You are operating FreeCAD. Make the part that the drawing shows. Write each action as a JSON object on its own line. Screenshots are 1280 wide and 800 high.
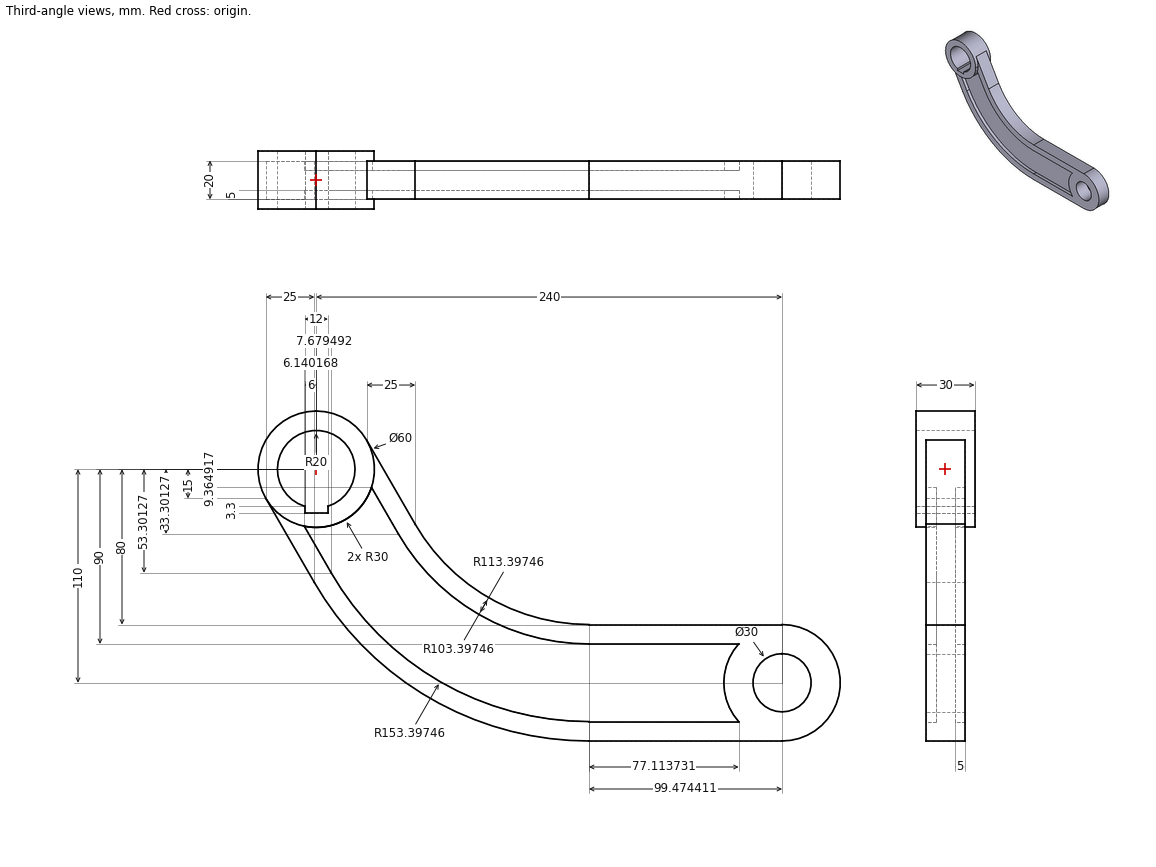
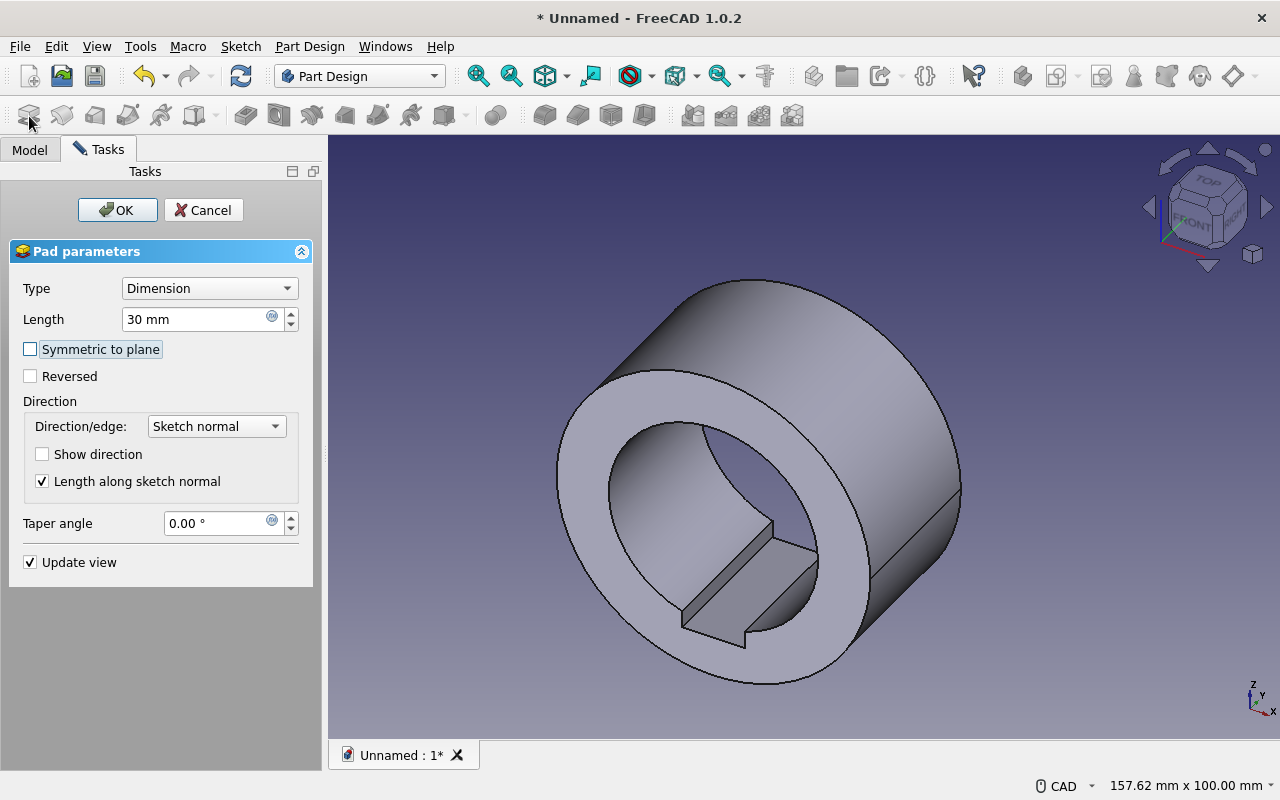
{"action": "left_click", "coordinate": [31, 349]}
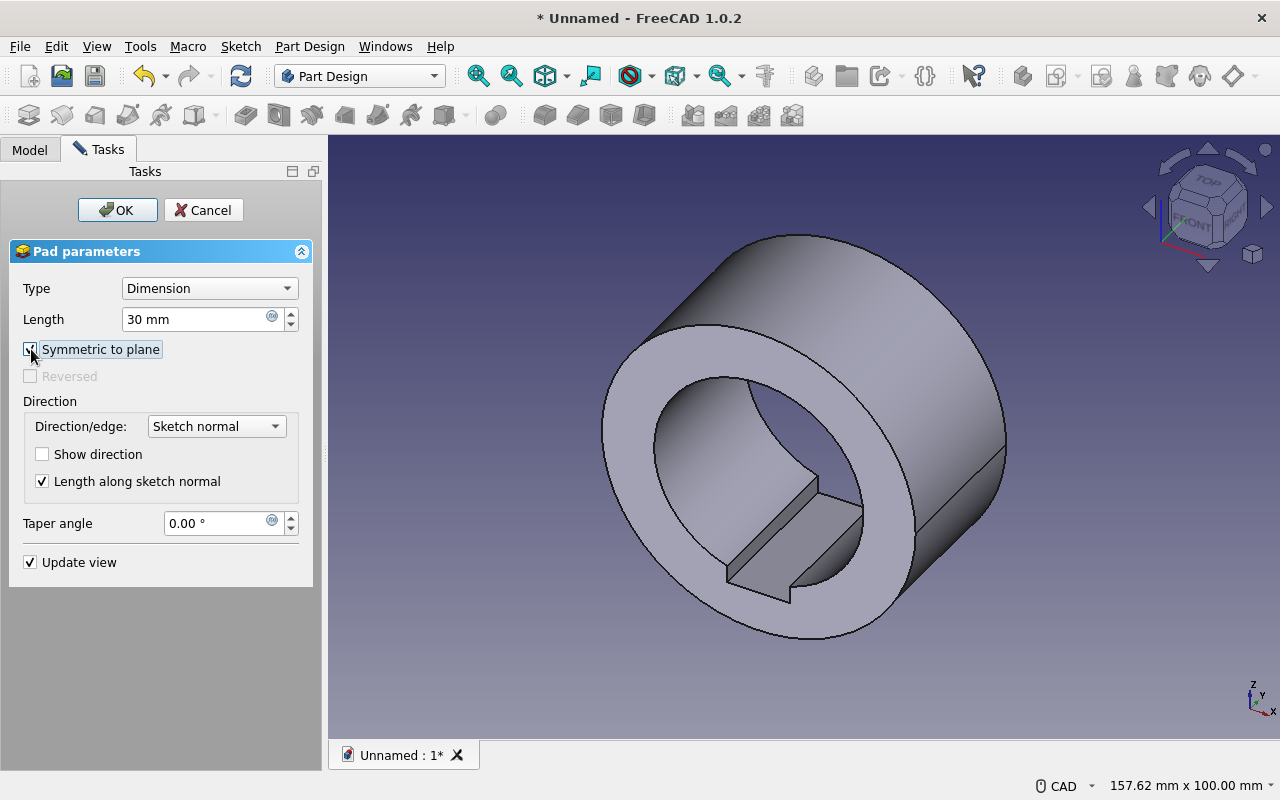
{"action": "left_click", "coordinate": [118, 210]}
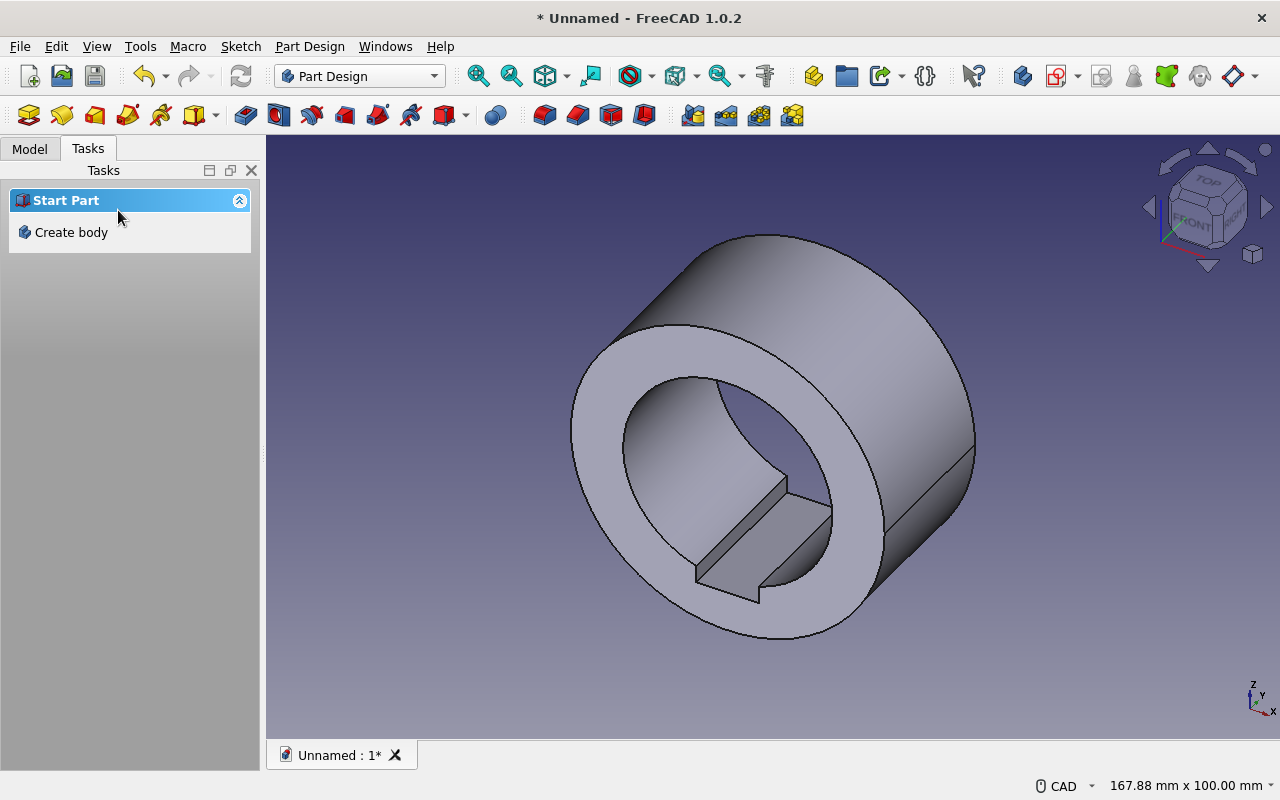
{"action": "left_click", "coordinate": [1056, 76]}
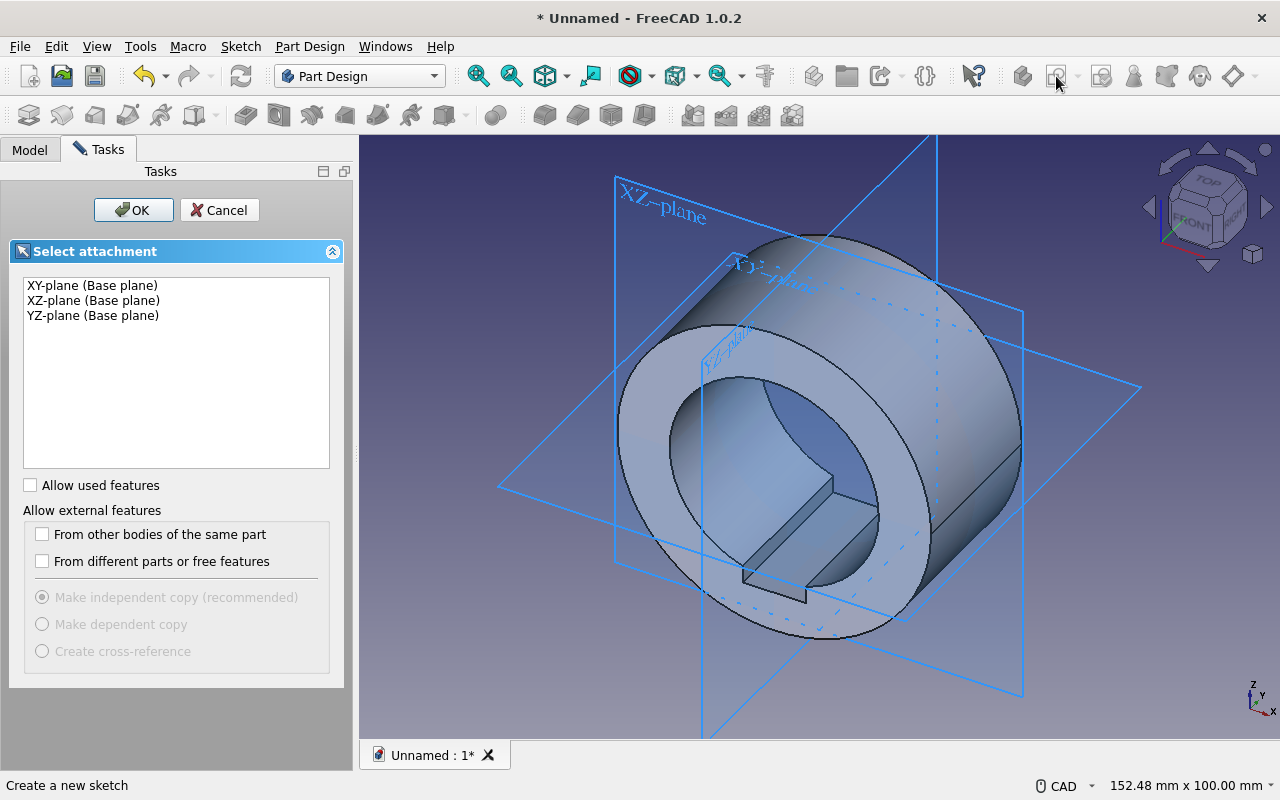
{"action": "left_click", "coordinate": [84, 300]}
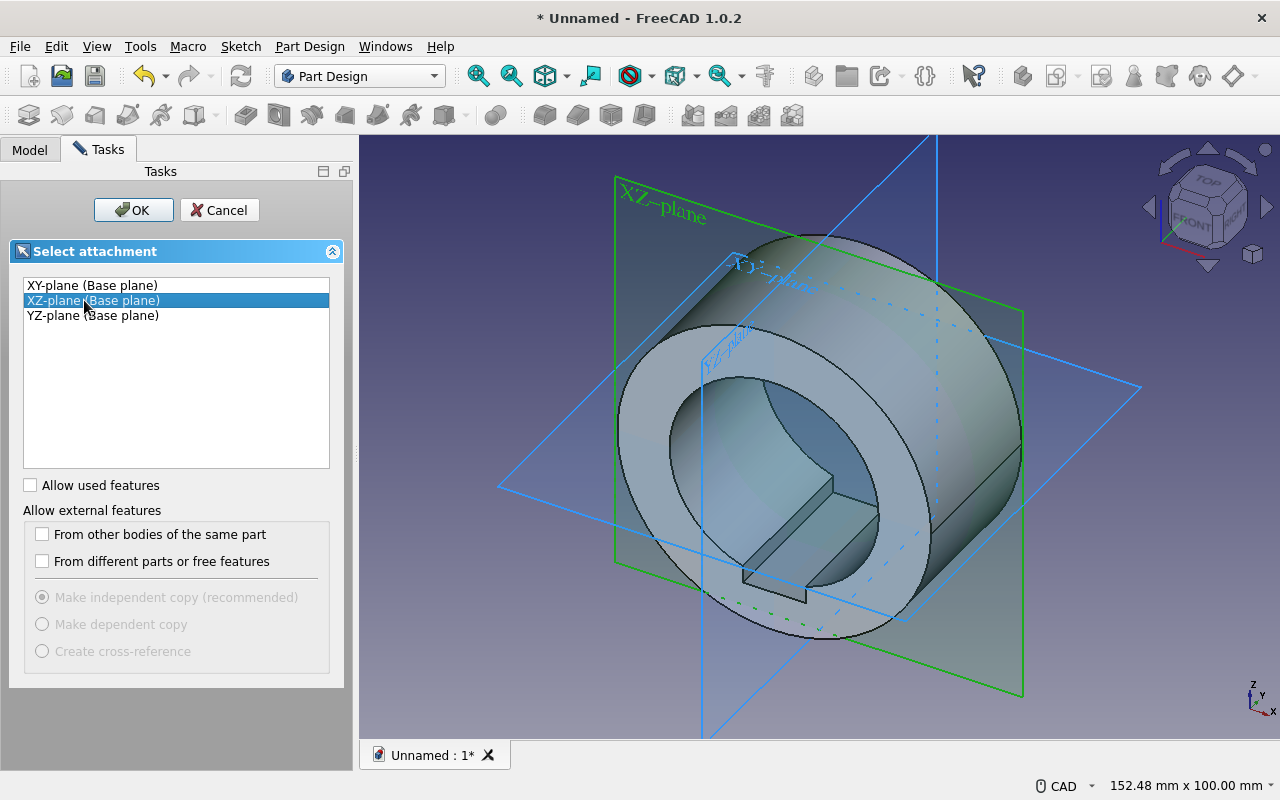
{"action": "left_click", "coordinate": [134, 210]}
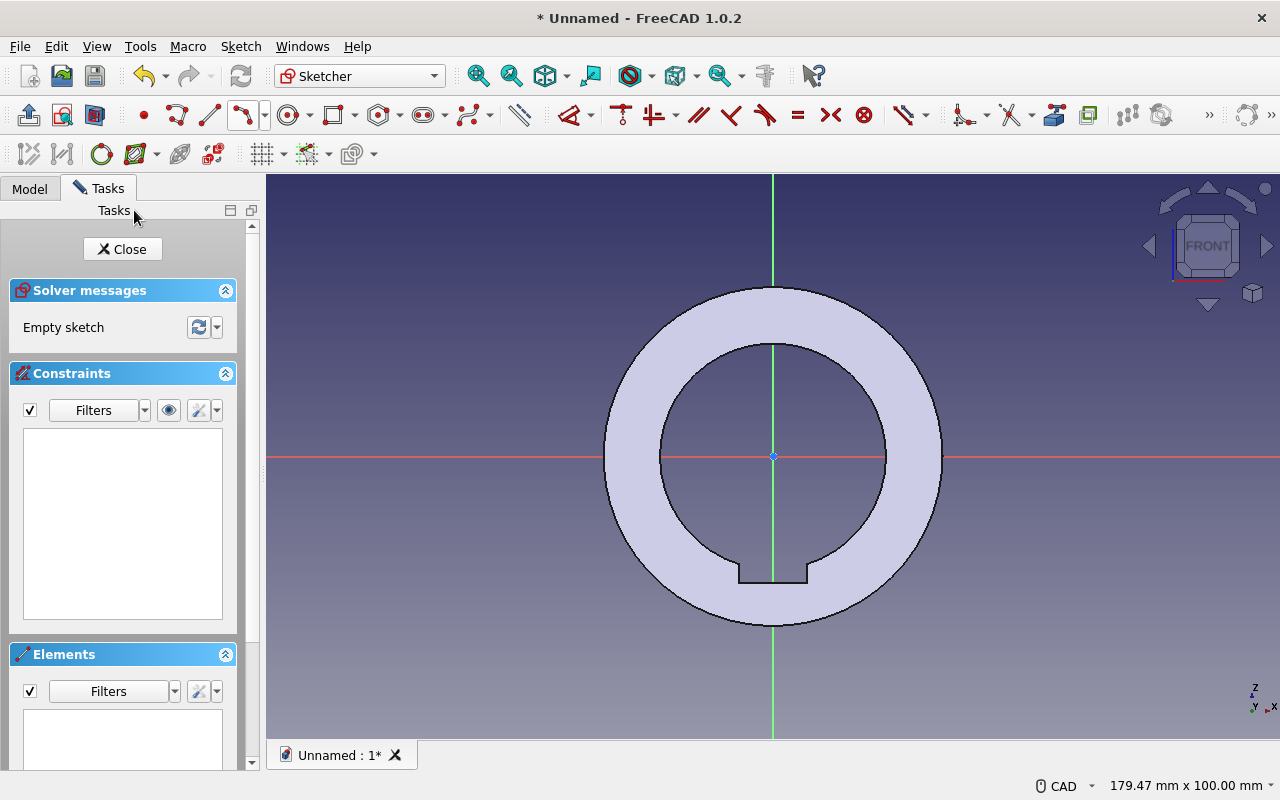
{"action": "left_click", "coordinate": [95, 116]}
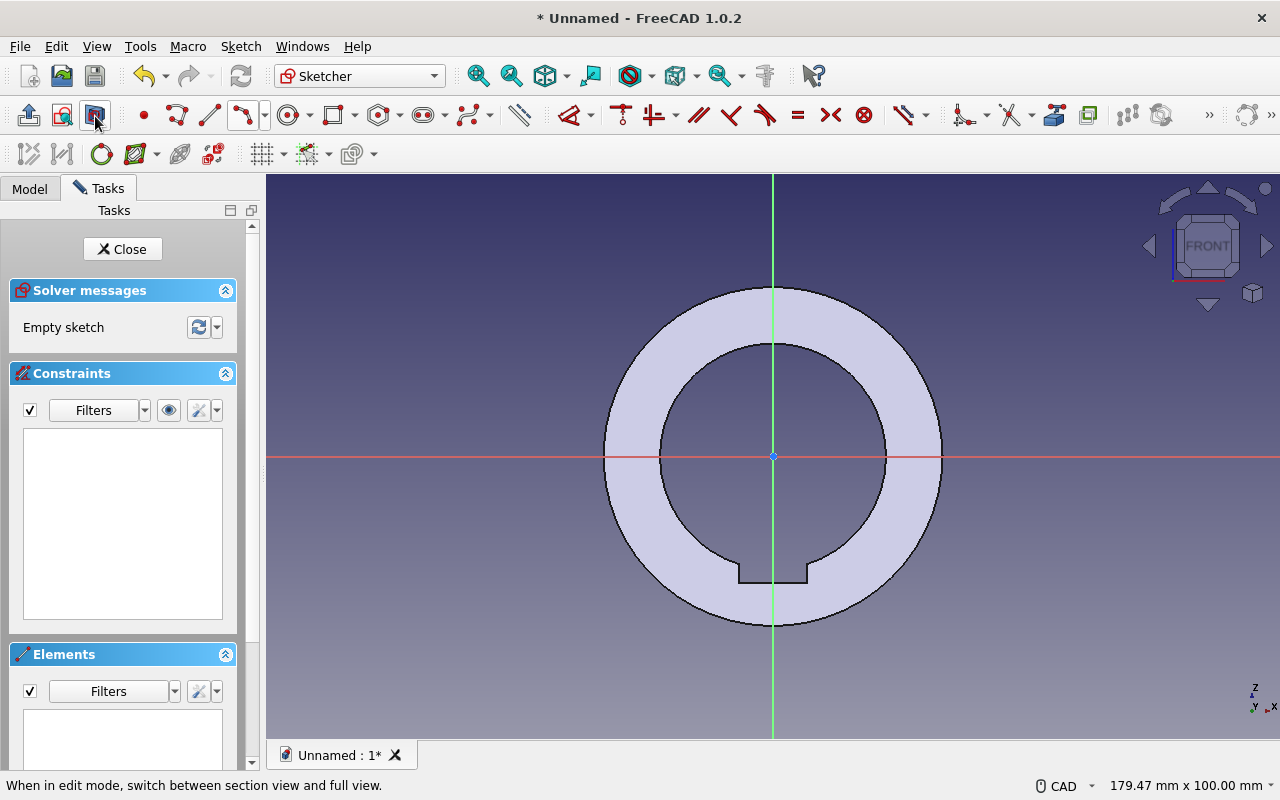
{"action": "scroll", "coordinate": [294, 251], "scroll_direction": "down", "scroll_amount": 5}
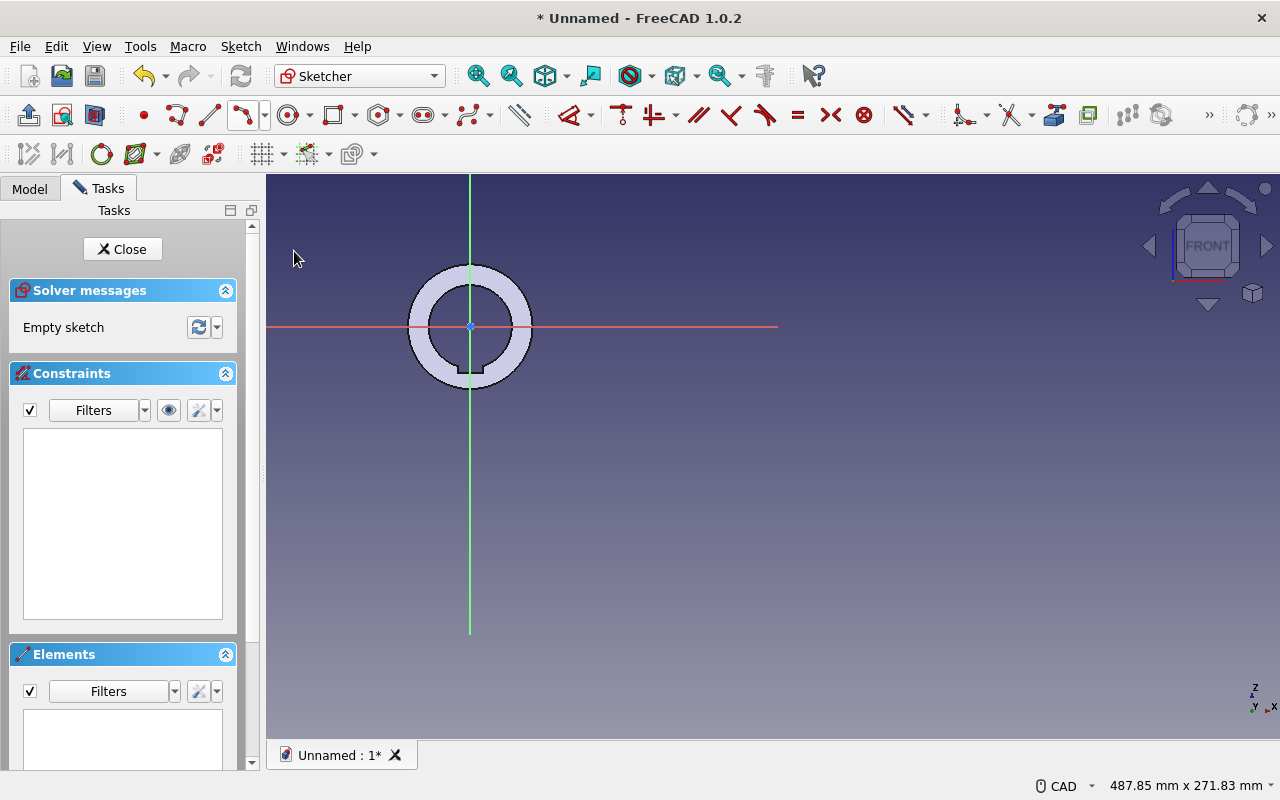
{"action": "left_click", "coordinate": [210, 116]}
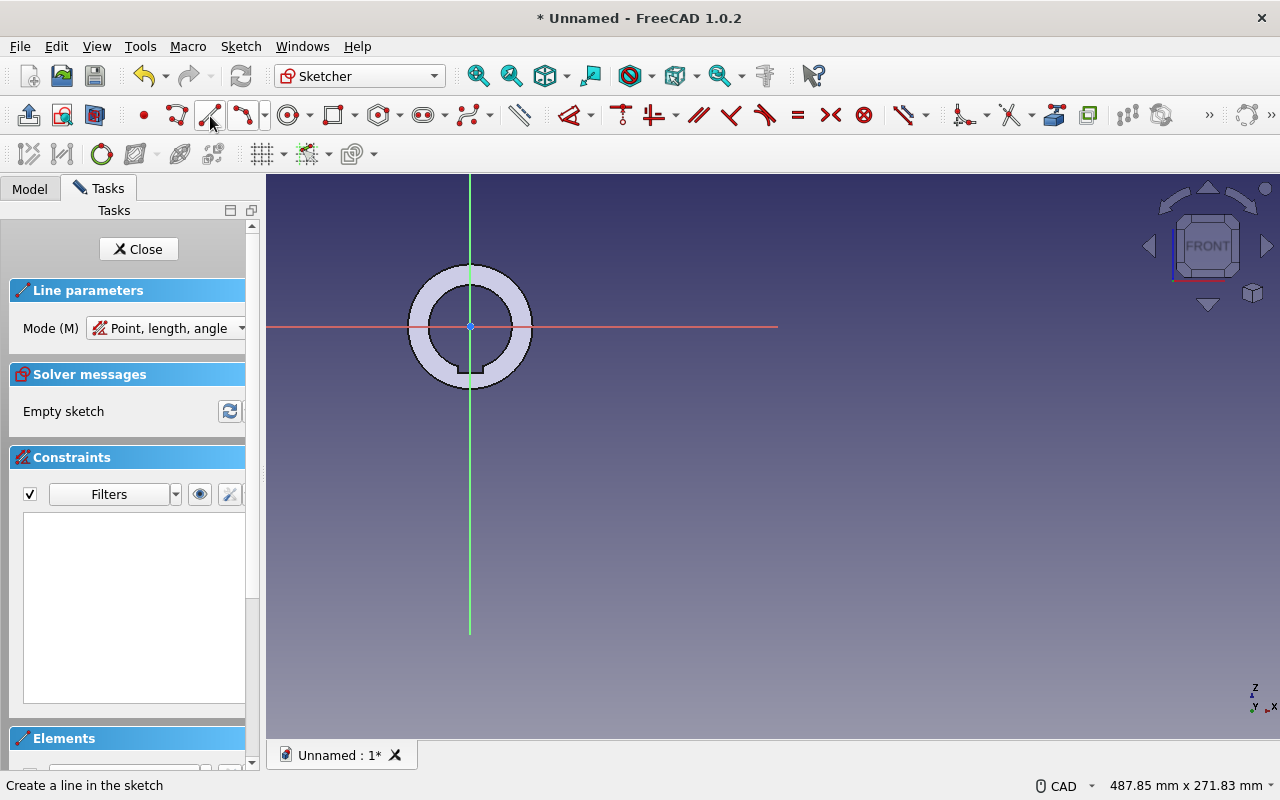
{"action": "scroll", "coordinate": [468, 448], "scroll_direction": "up", "scroll_amount": 11}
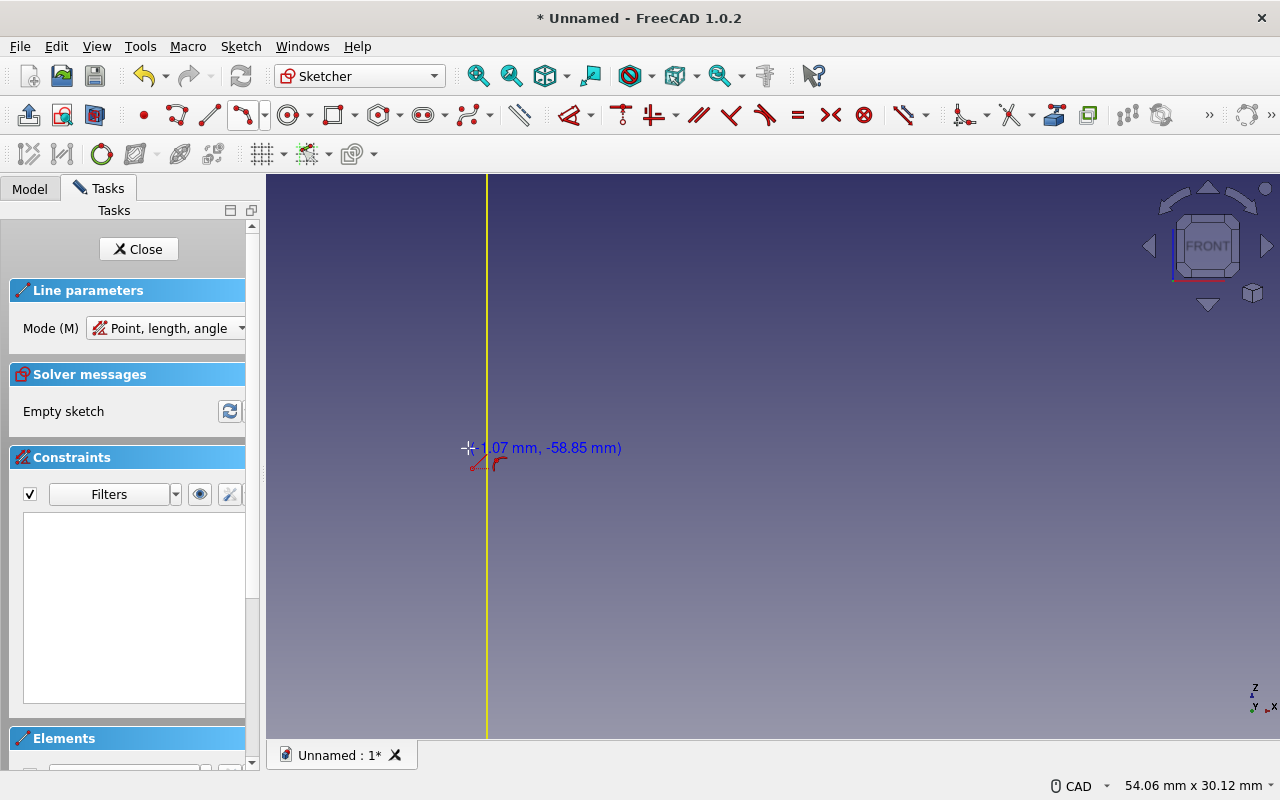
{"action": "left_click", "coordinate": [468, 443]}